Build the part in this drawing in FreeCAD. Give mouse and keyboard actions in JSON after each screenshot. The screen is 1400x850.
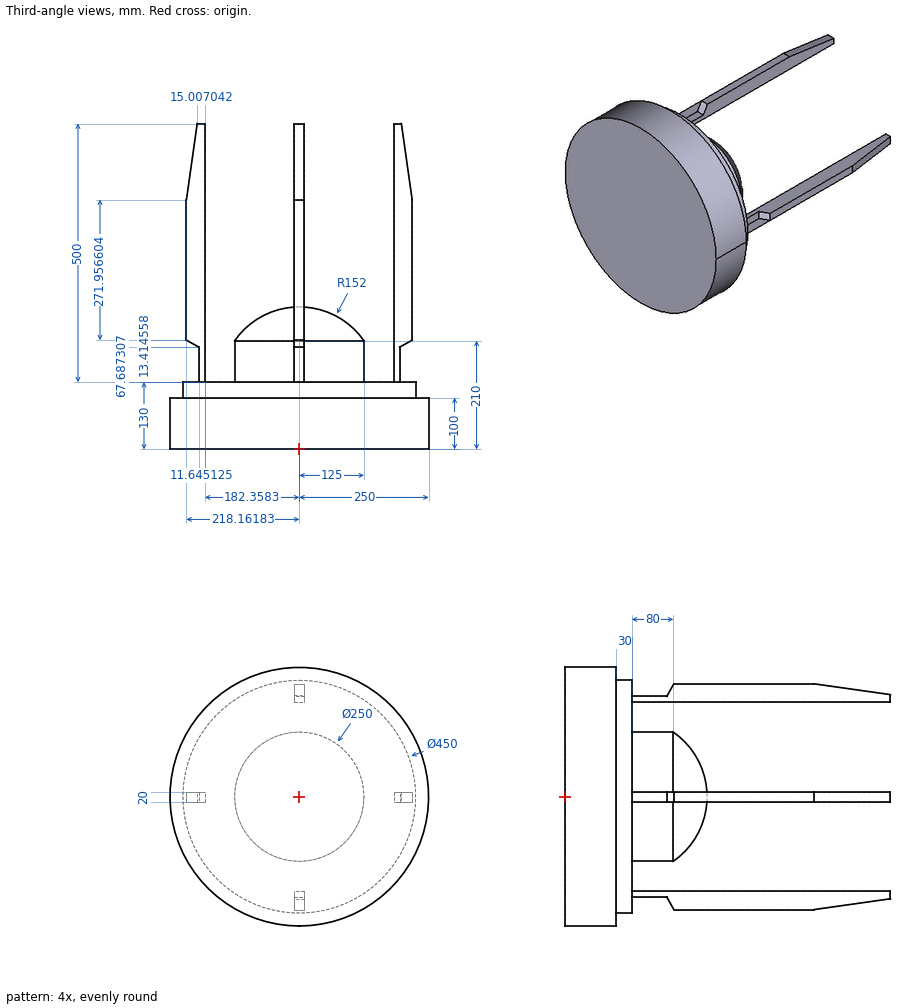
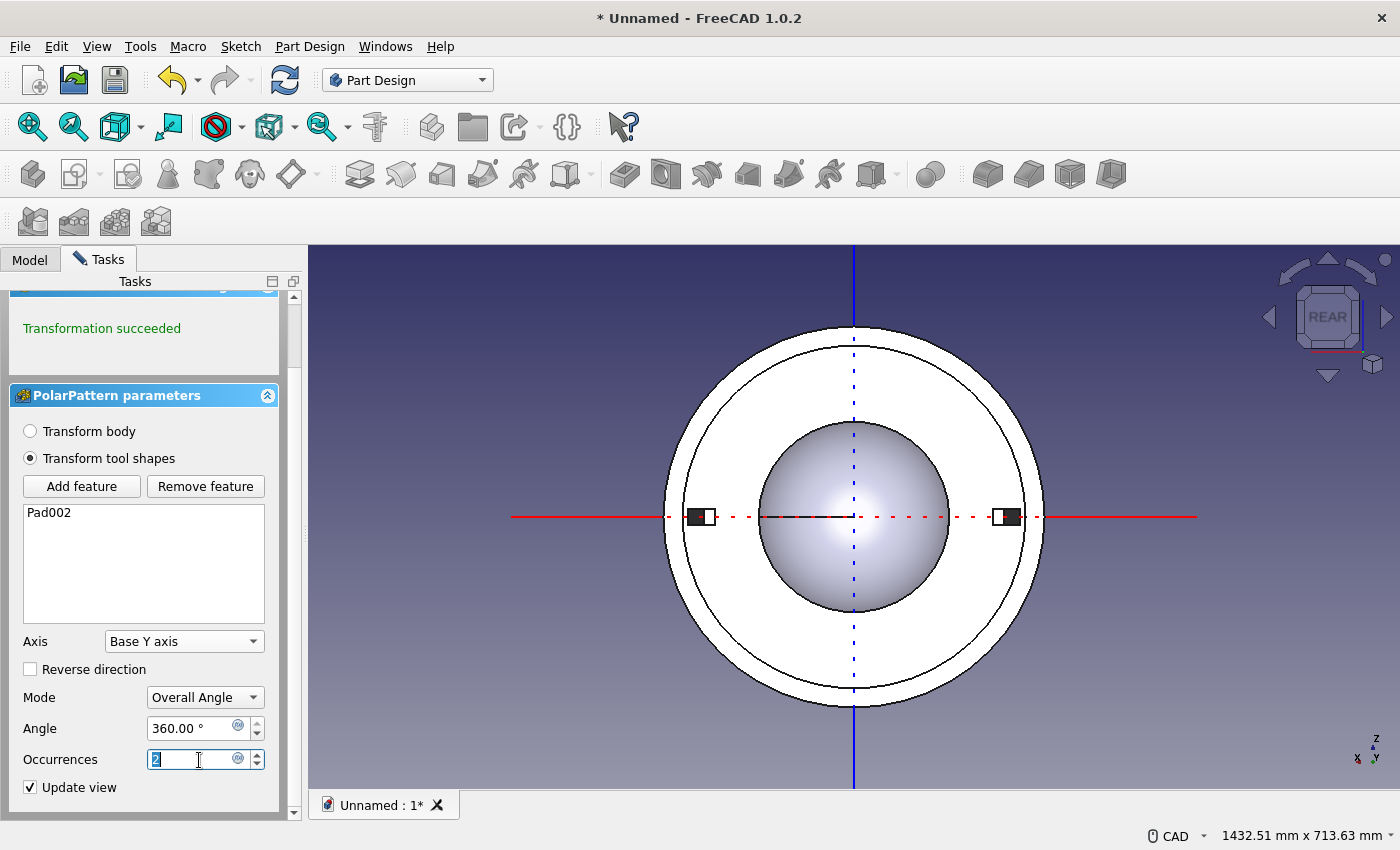
{"action": "type", "text": "4"}
{"action": "key", "text": "Tab"}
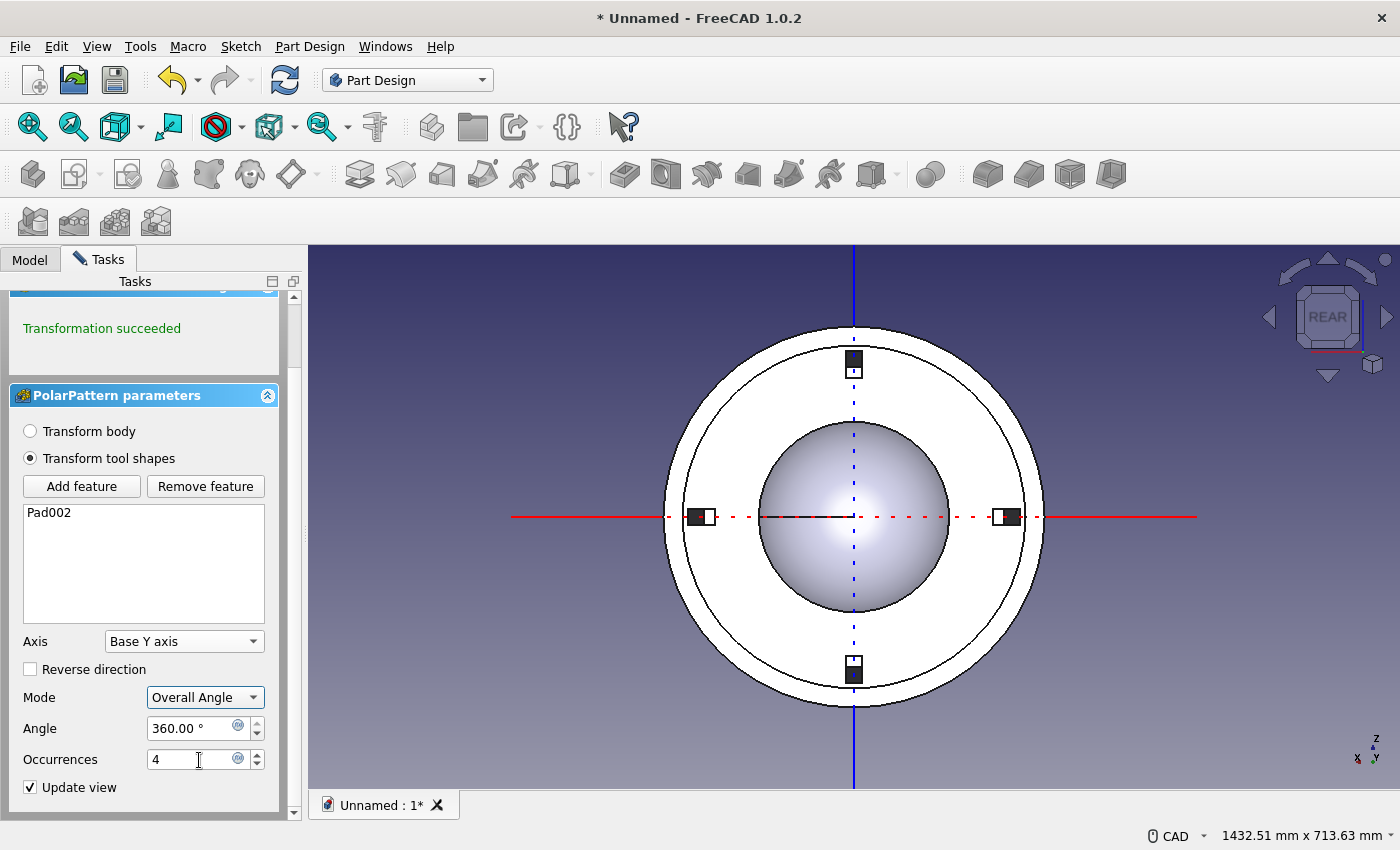
{"action": "scroll", "coordinate": [294, 556], "scroll_direction": "up", "scroll_amount": 3}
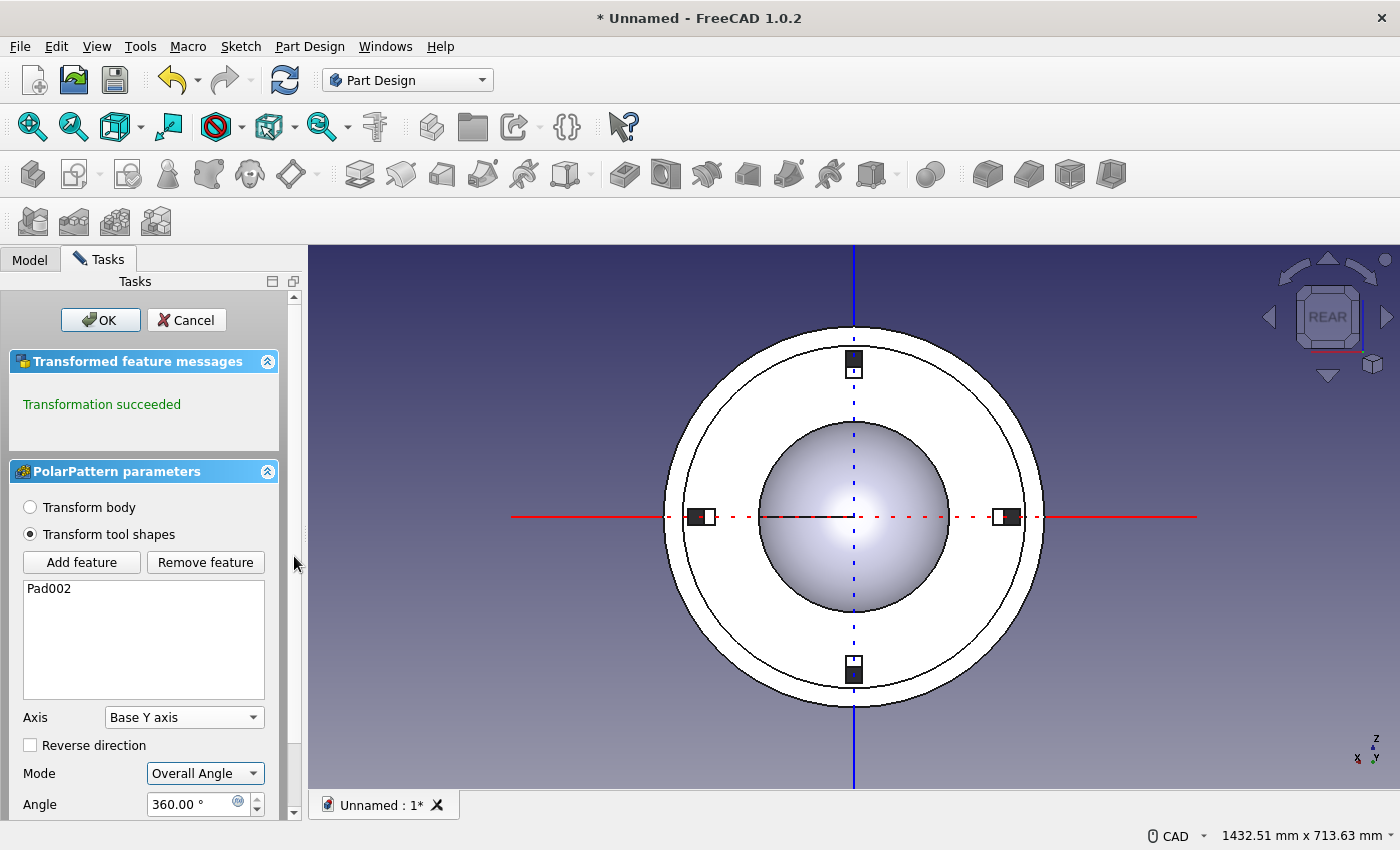
{"action": "left_click", "coordinate": [101, 320]}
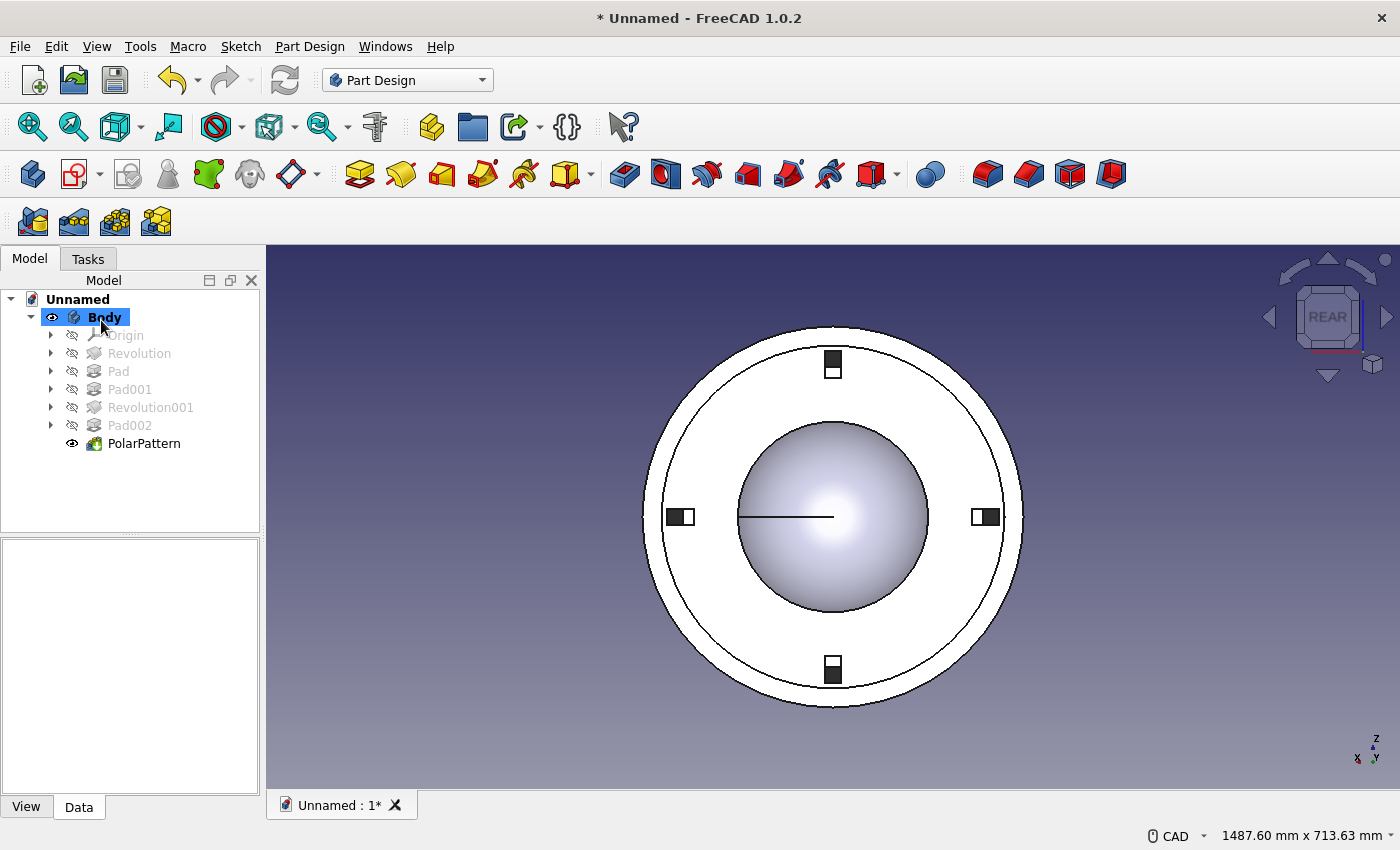
{"action": "key", "text": "0"}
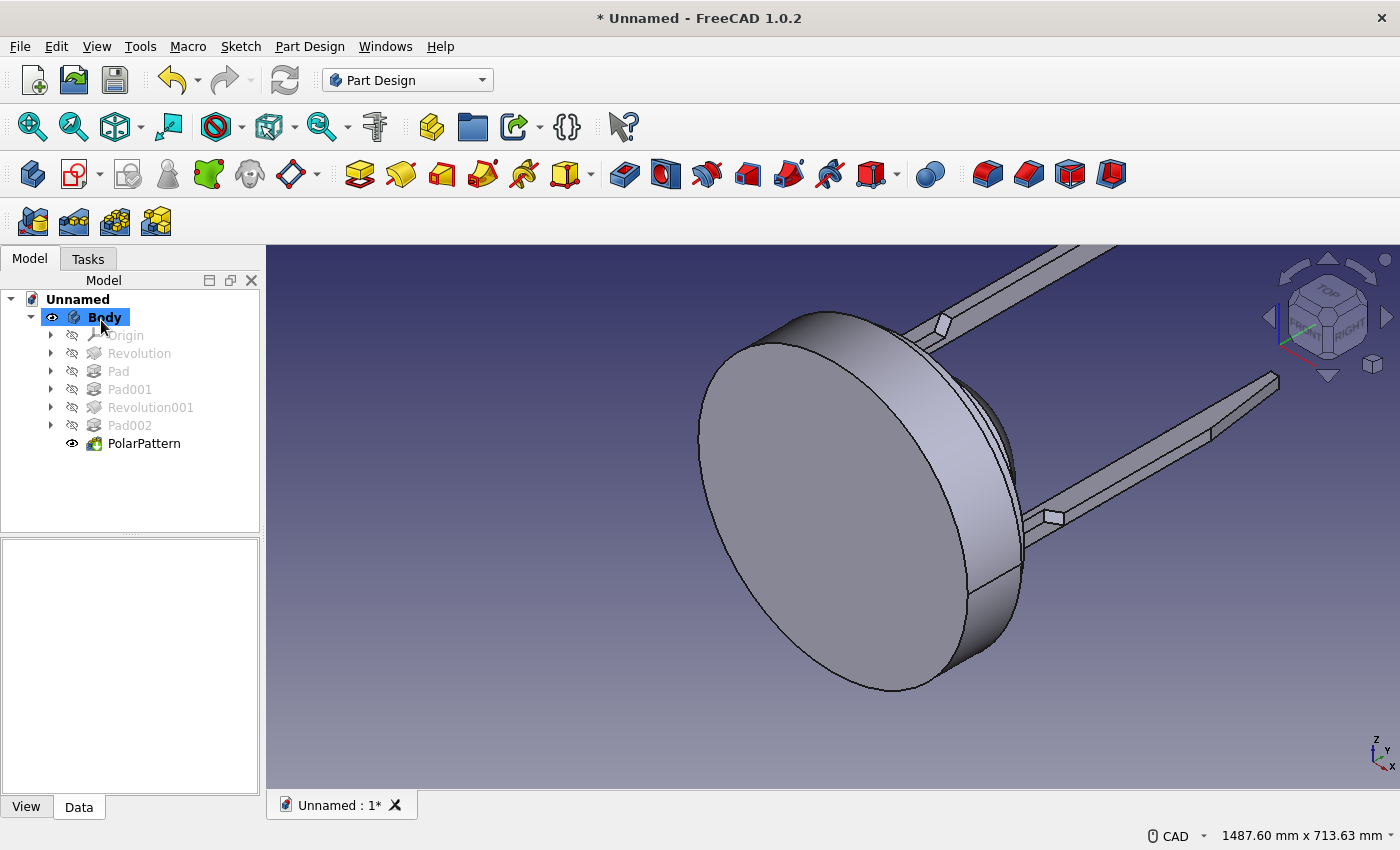
{"action": "left_click", "coordinate": [33, 128]}